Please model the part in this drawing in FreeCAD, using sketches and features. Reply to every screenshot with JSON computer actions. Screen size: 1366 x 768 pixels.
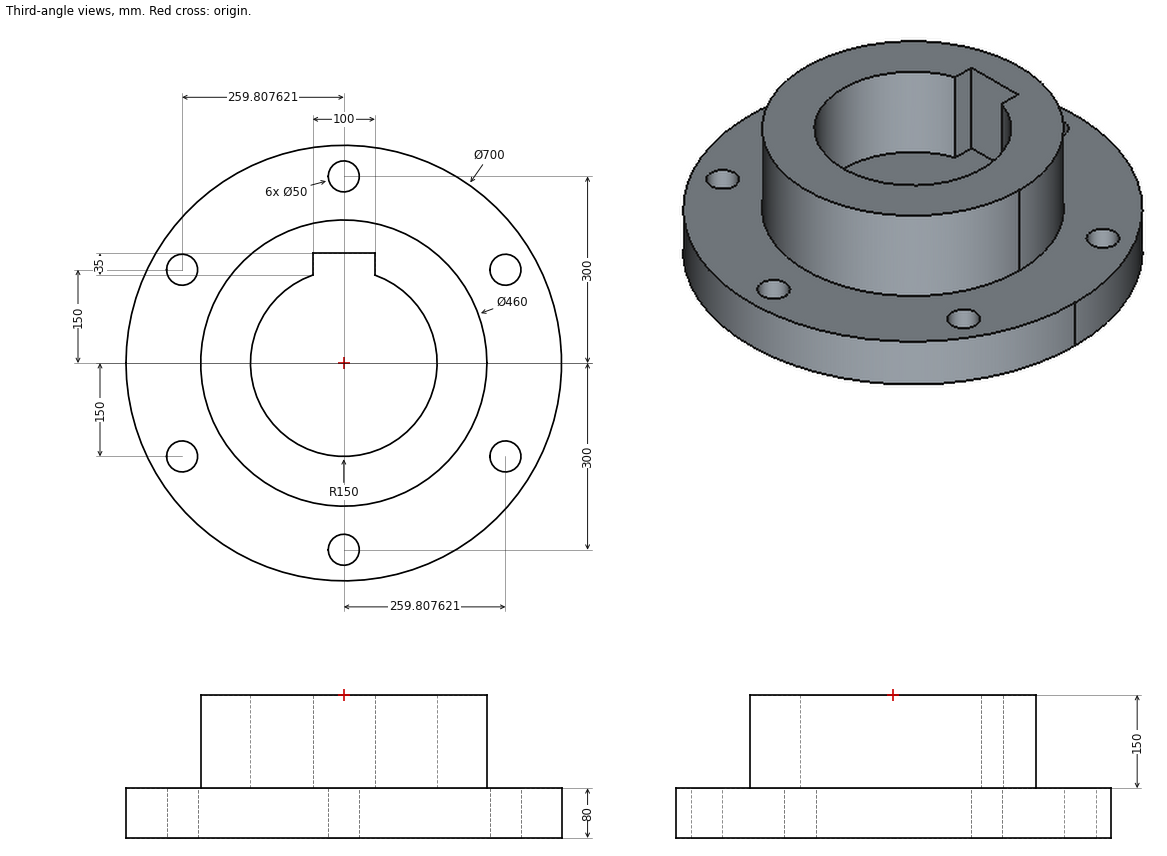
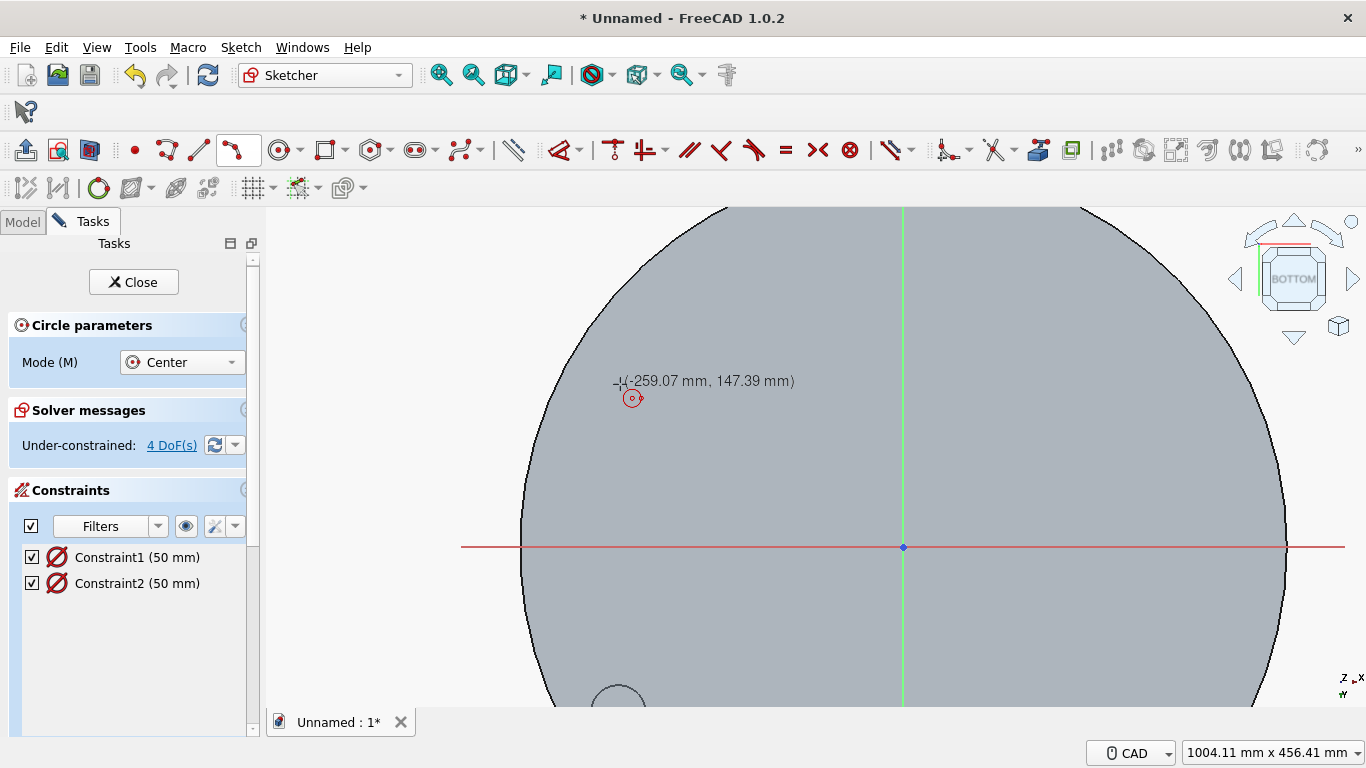
{"action": "left_click", "coordinate": [619, 383]}
{"action": "mouse_move", "coordinate": [638, 364]}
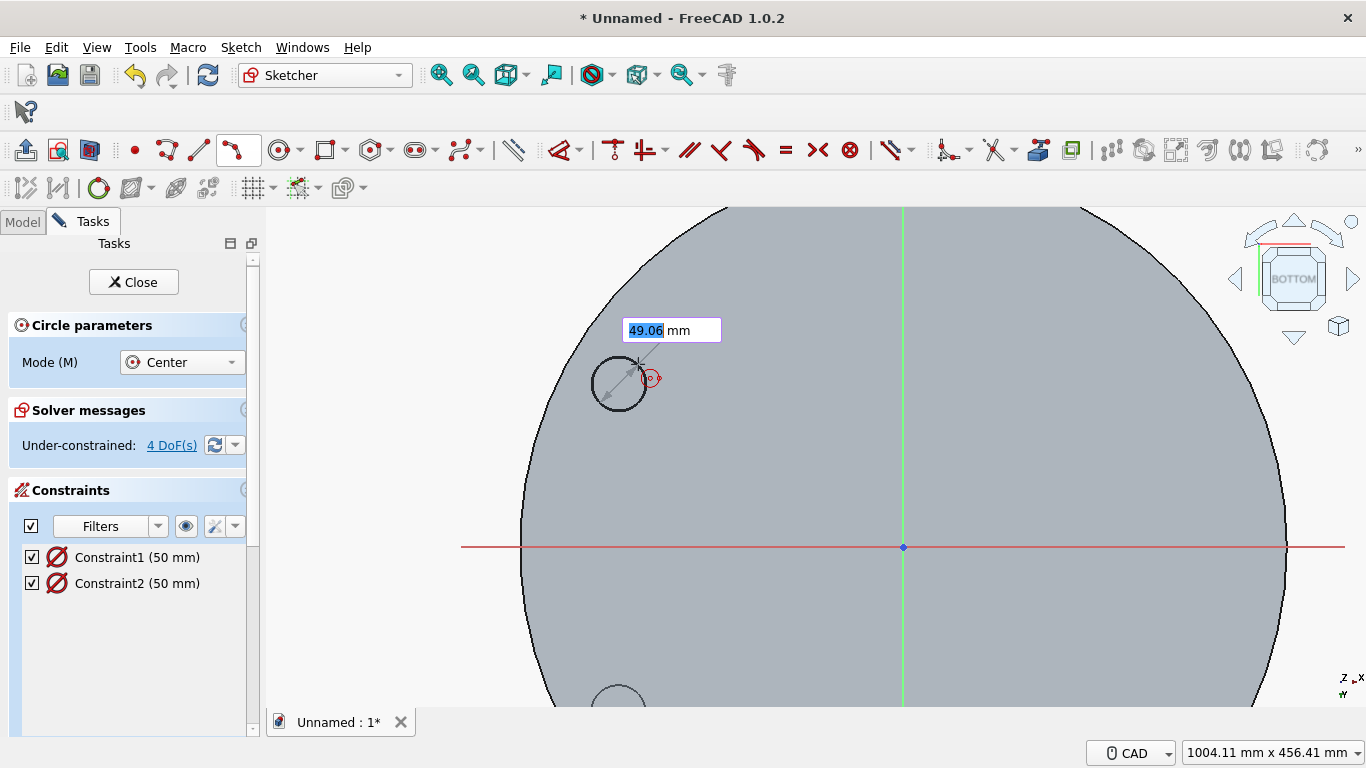
{"action": "type", "text": "50"}
{"action": "key", "text": "Return"}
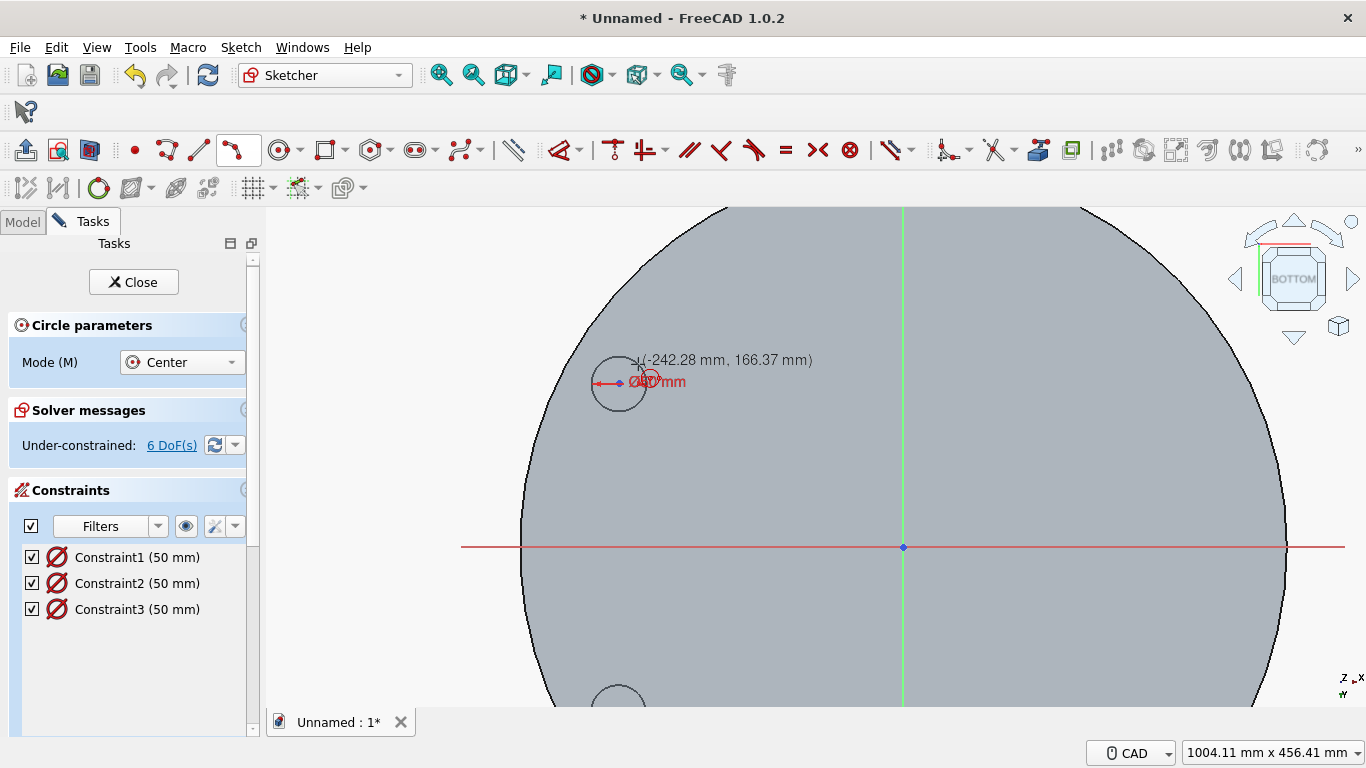
{"action": "scroll", "coordinate": [620, 383], "scroll_direction": "down", "scroll_amount": 4}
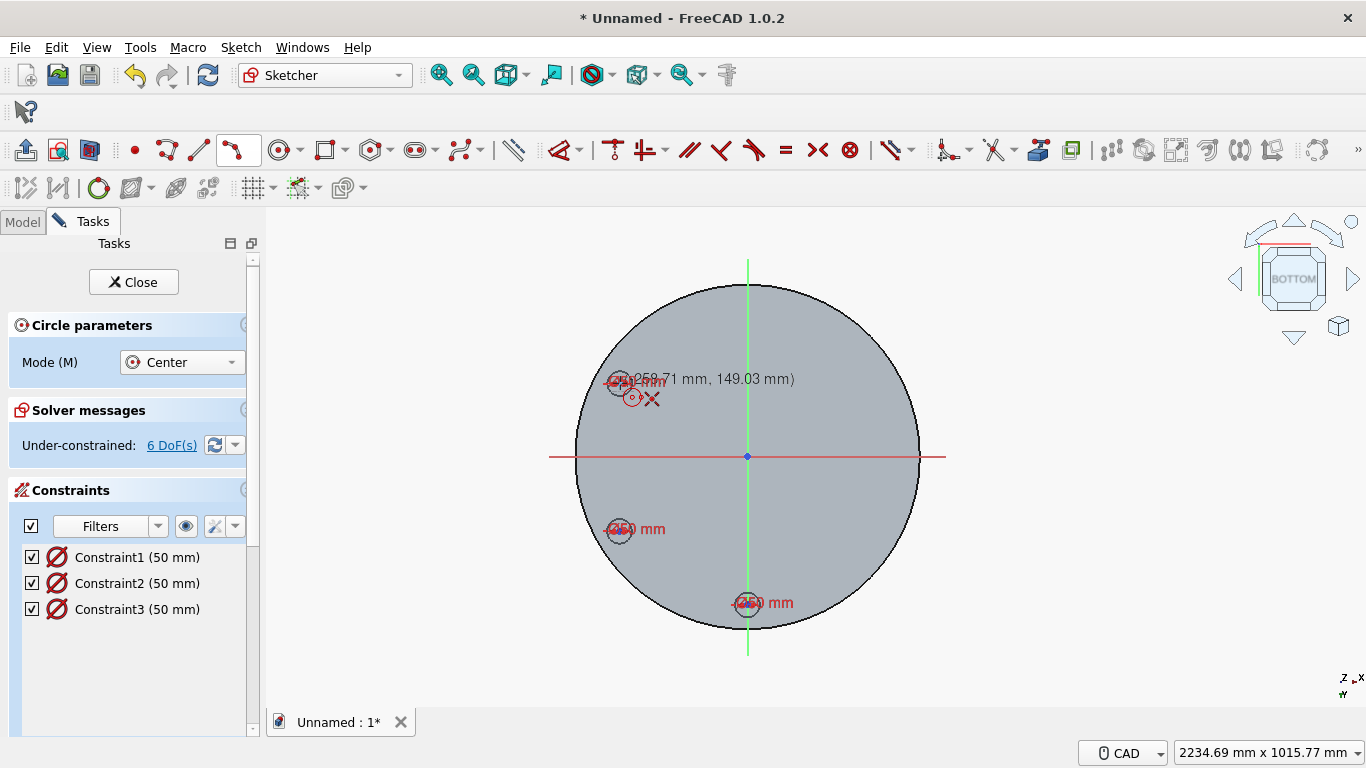
{"action": "scroll", "coordinate": [748, 309], "scroll_direction": "up", "scroll_amount": 4}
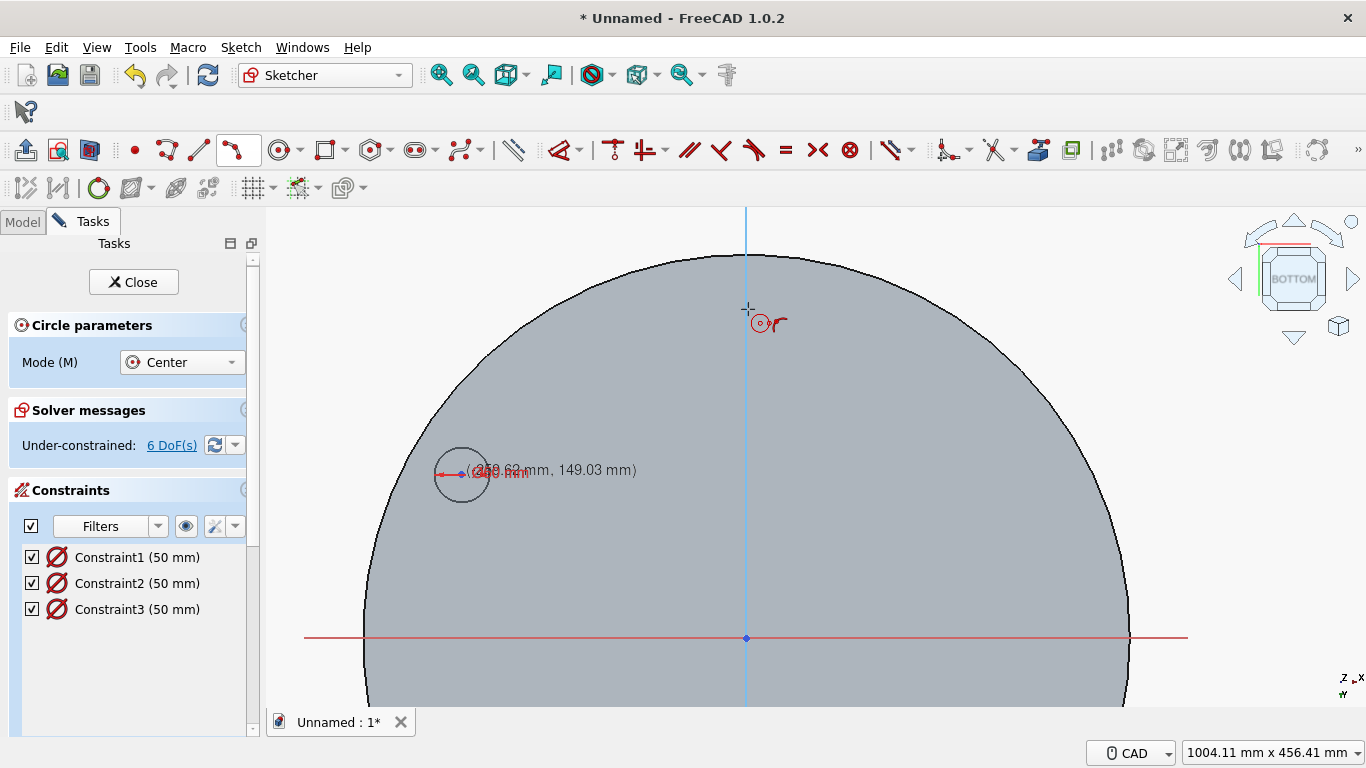
{"action": "left_click", "coordinate": [746, 309]}
{"action": "mouse_move", "coordinate": [766, 290]}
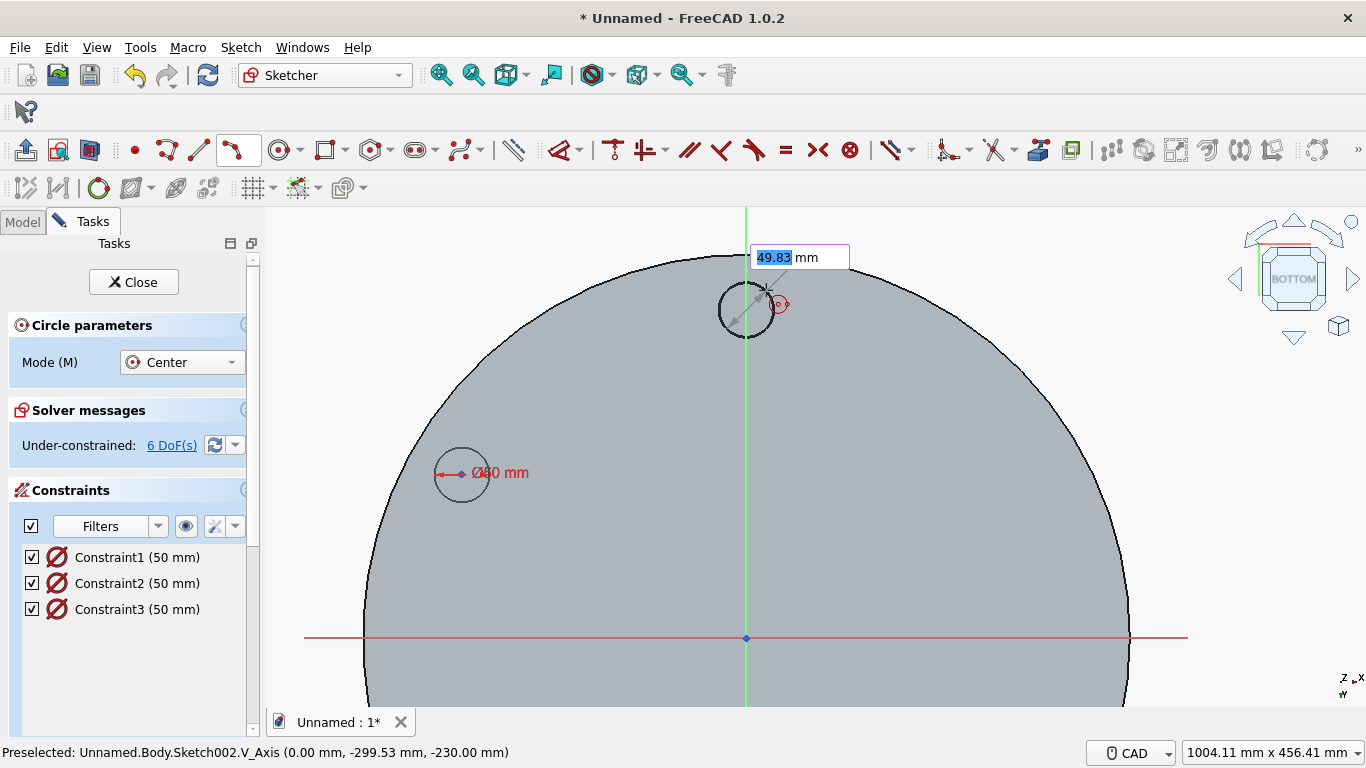
{"action": "type", "text": "50"}
{"action": "key", "text": "Return"}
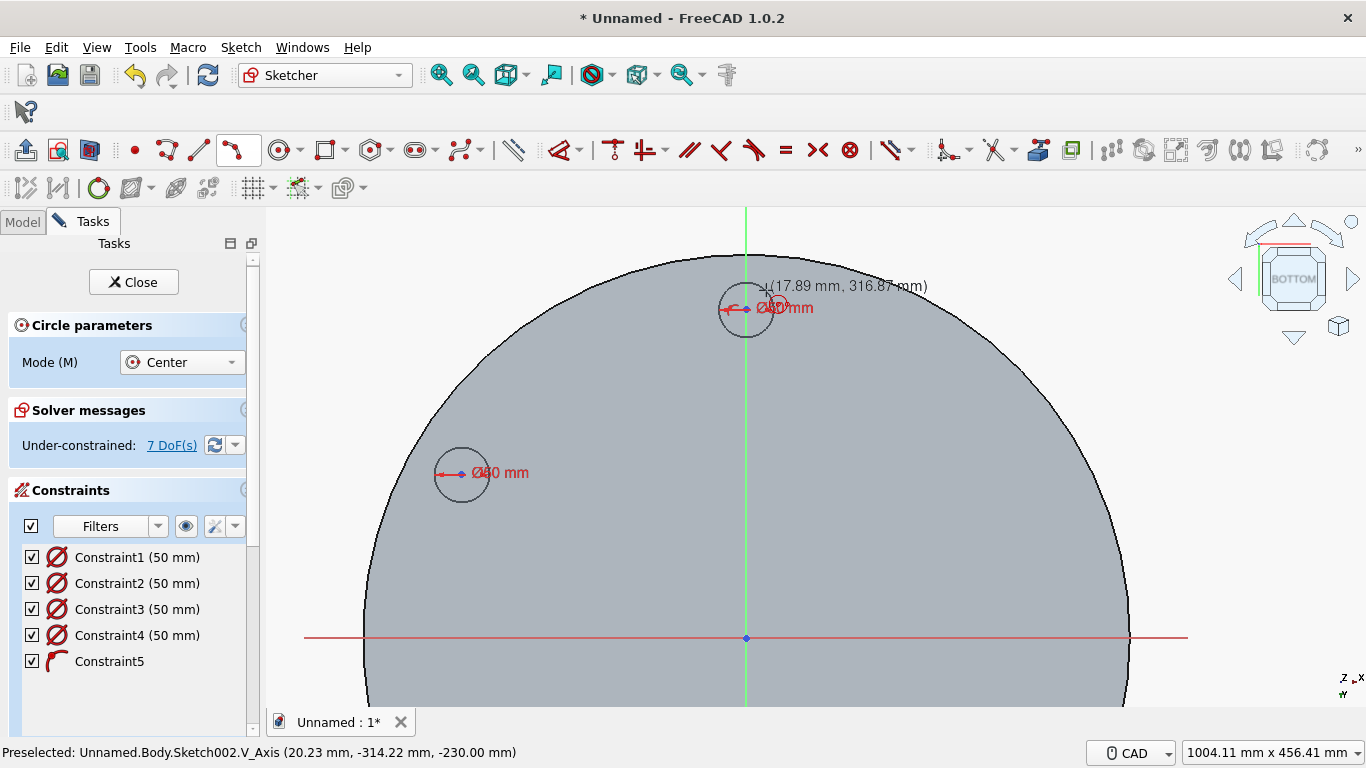
{"action": "left_click", "coordinate": [1031, 474]}
{"action": "mouse_move", "coordinate": [1050, 454]}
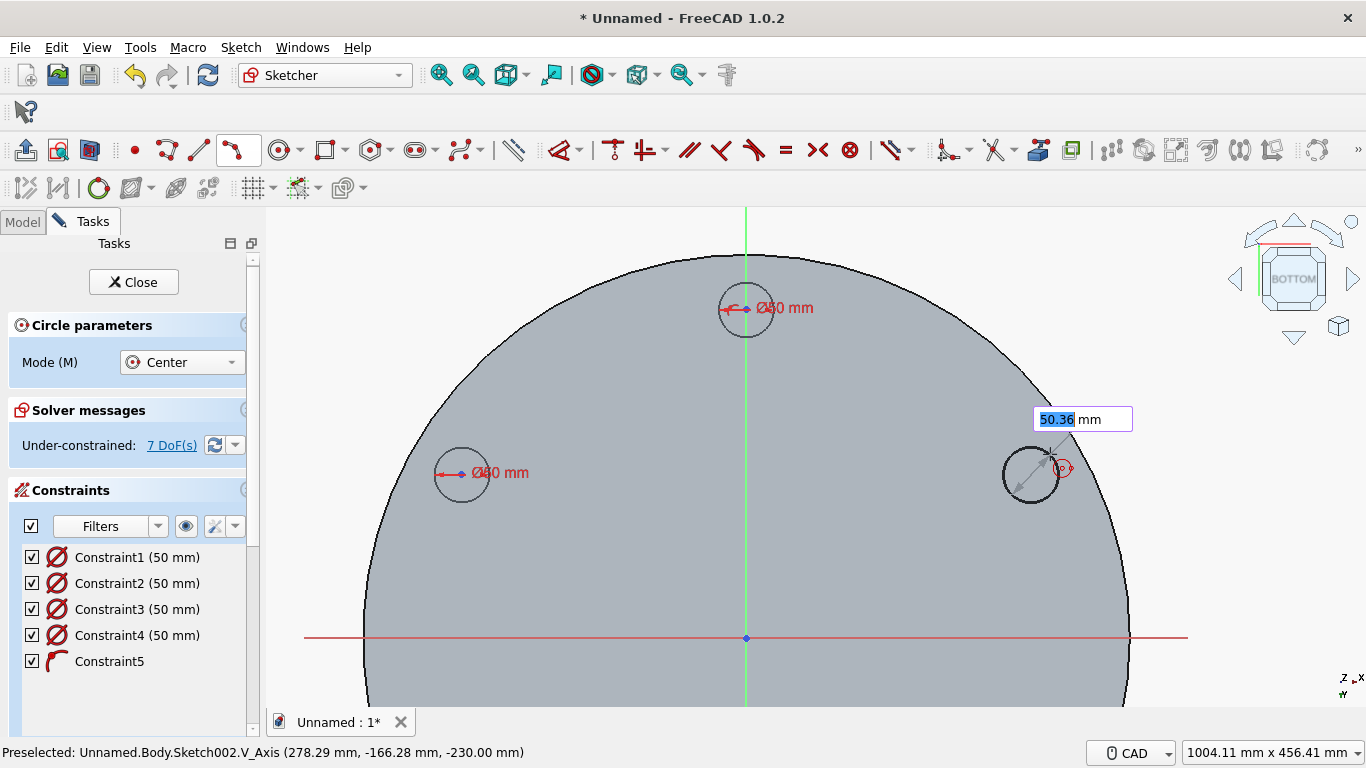
{"action": "type", "text": "50"}
{"action": "key", "text": "Return"}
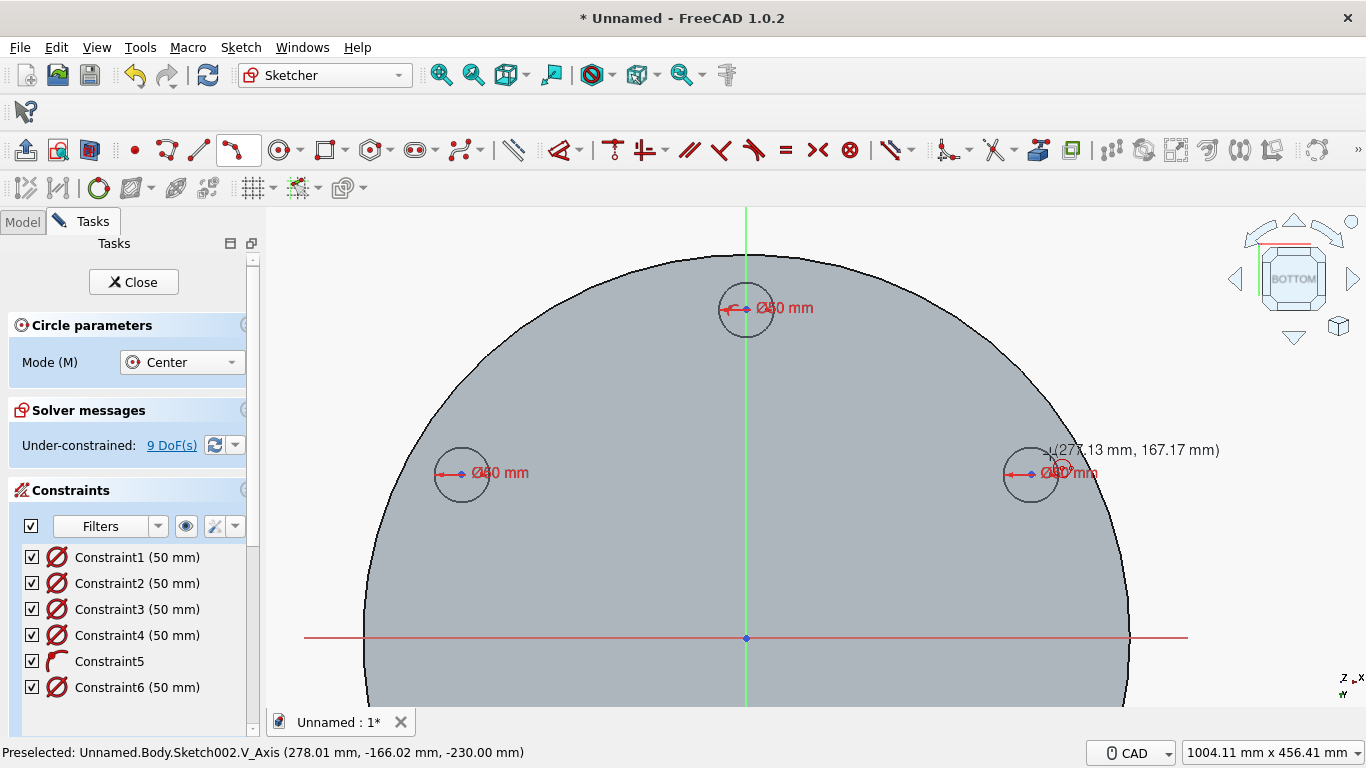
{"action": "scroll", "coordinate": [748, 309], "scroll_direction": "down", "scroll_amount": 4}